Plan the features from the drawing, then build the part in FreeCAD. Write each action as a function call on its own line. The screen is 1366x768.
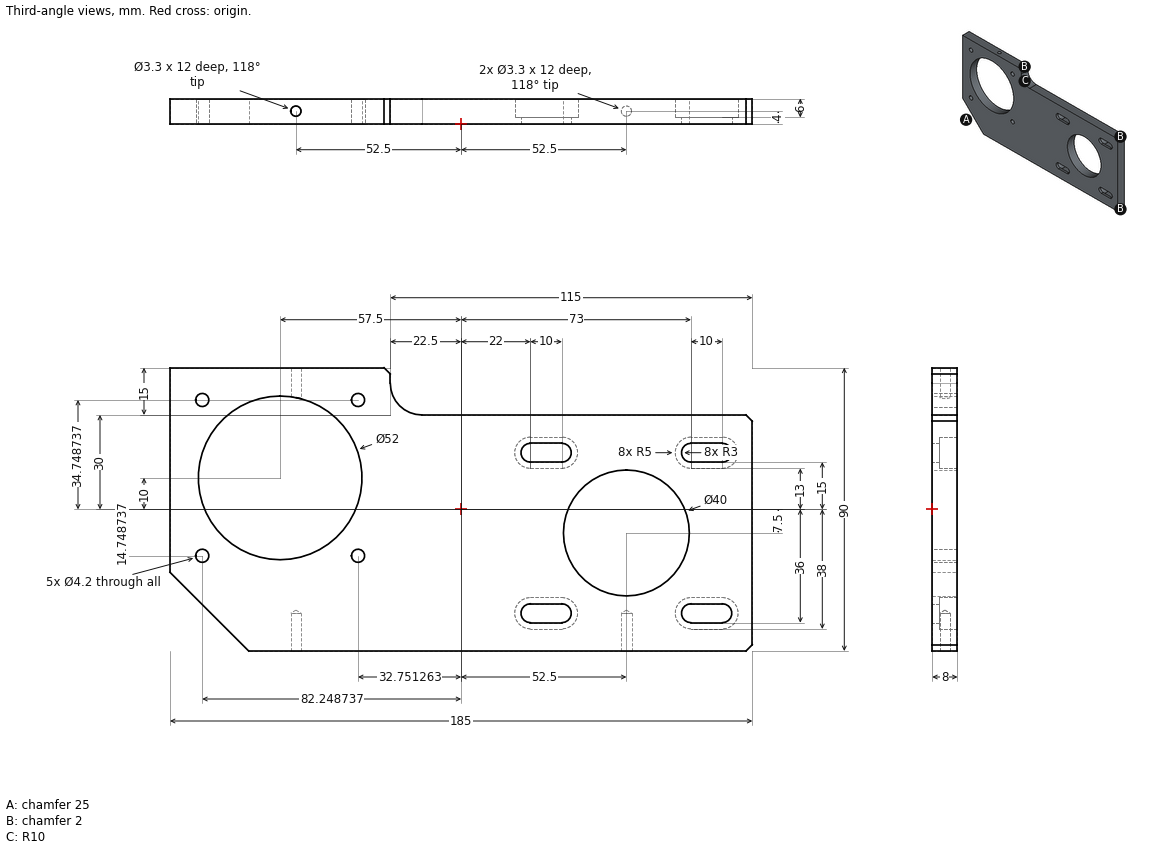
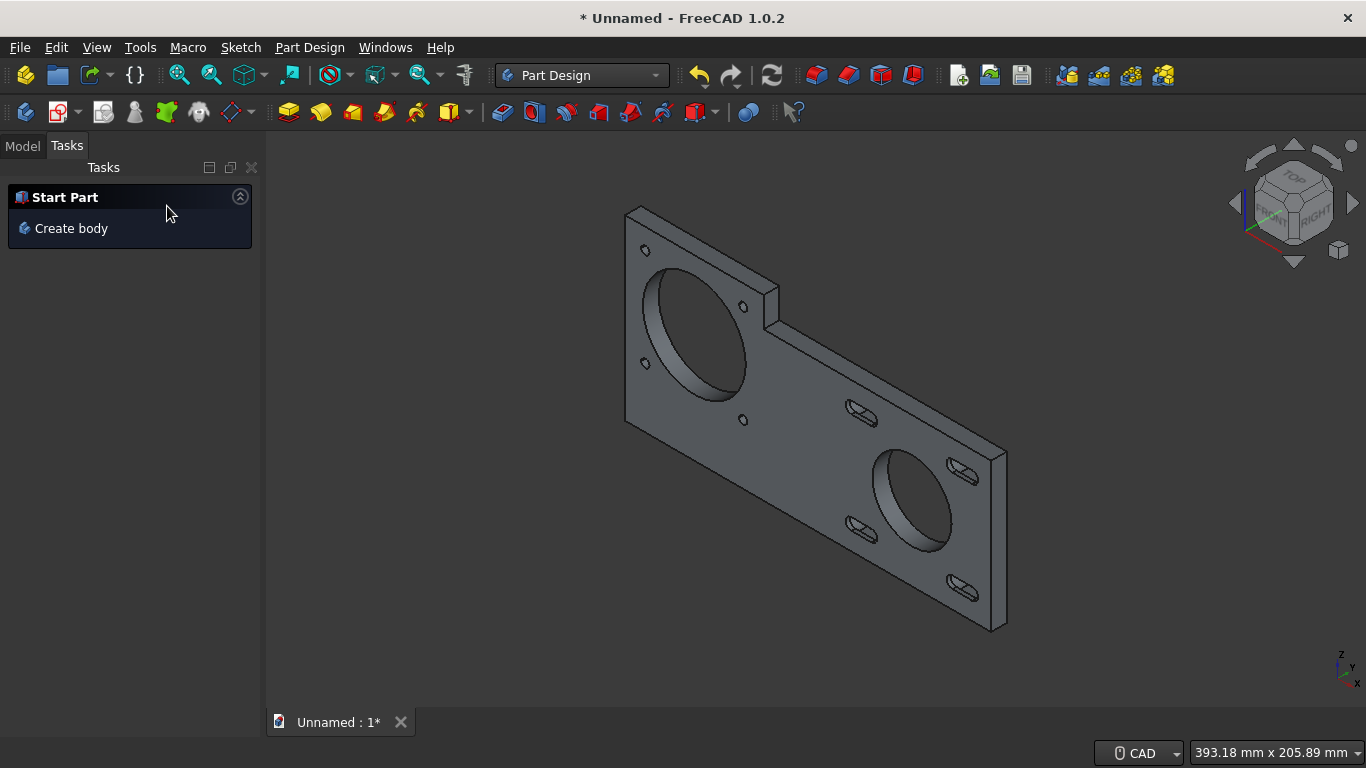
click(764, 282)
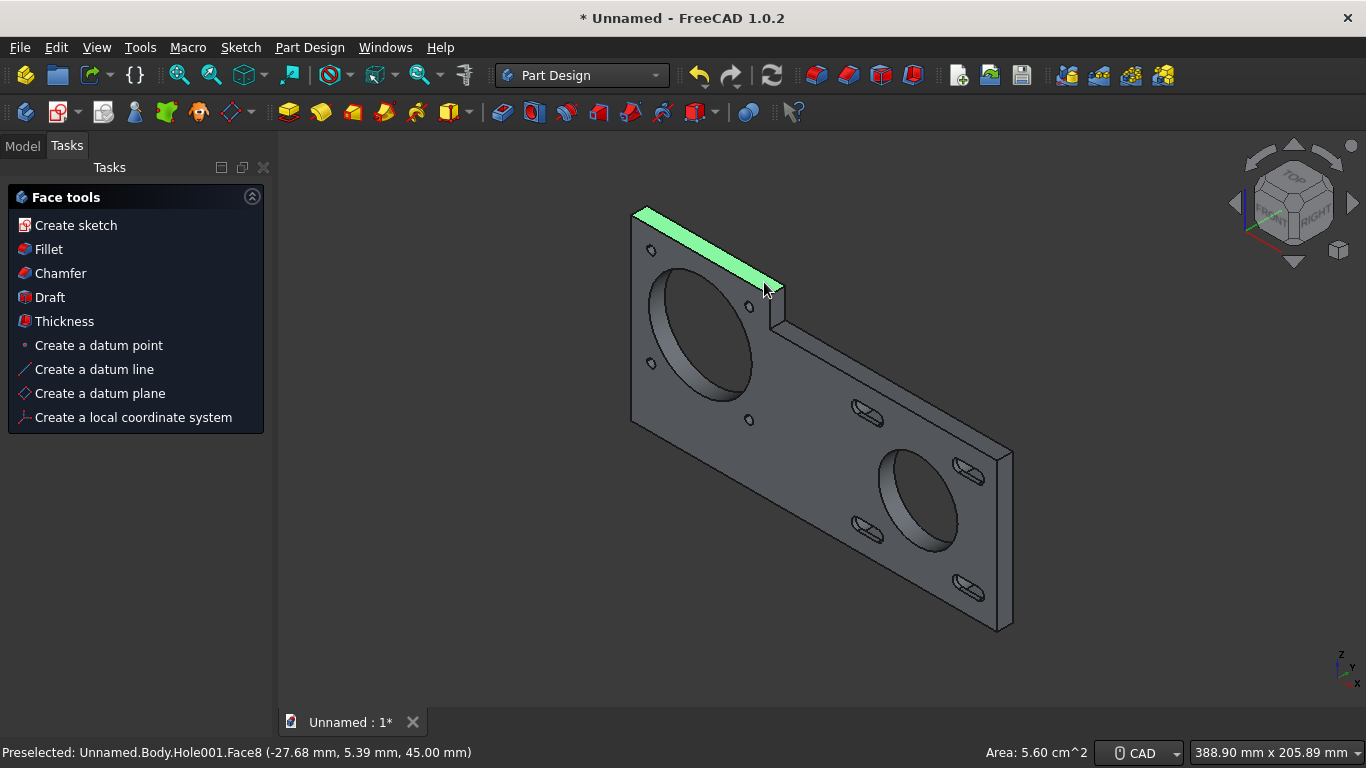
click(58, 112)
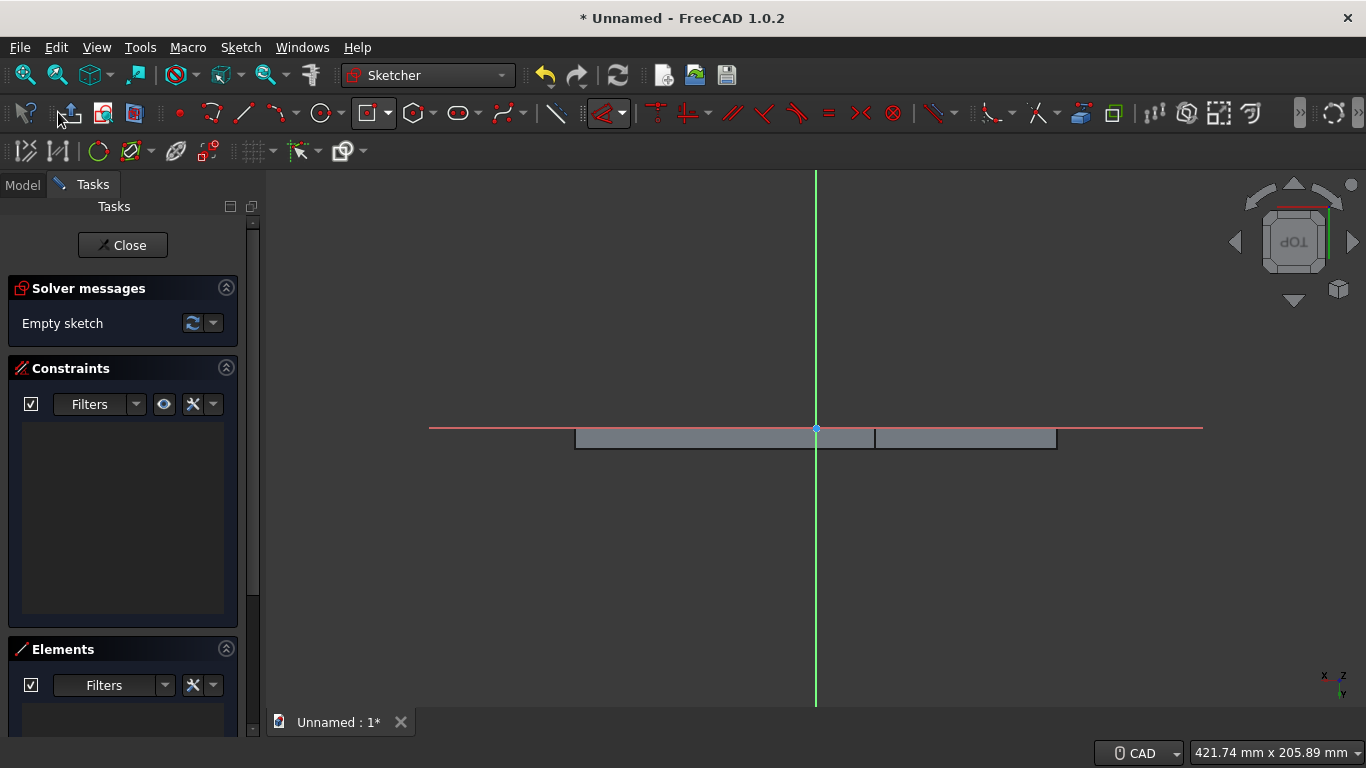
scroll(964, 439, up, 15)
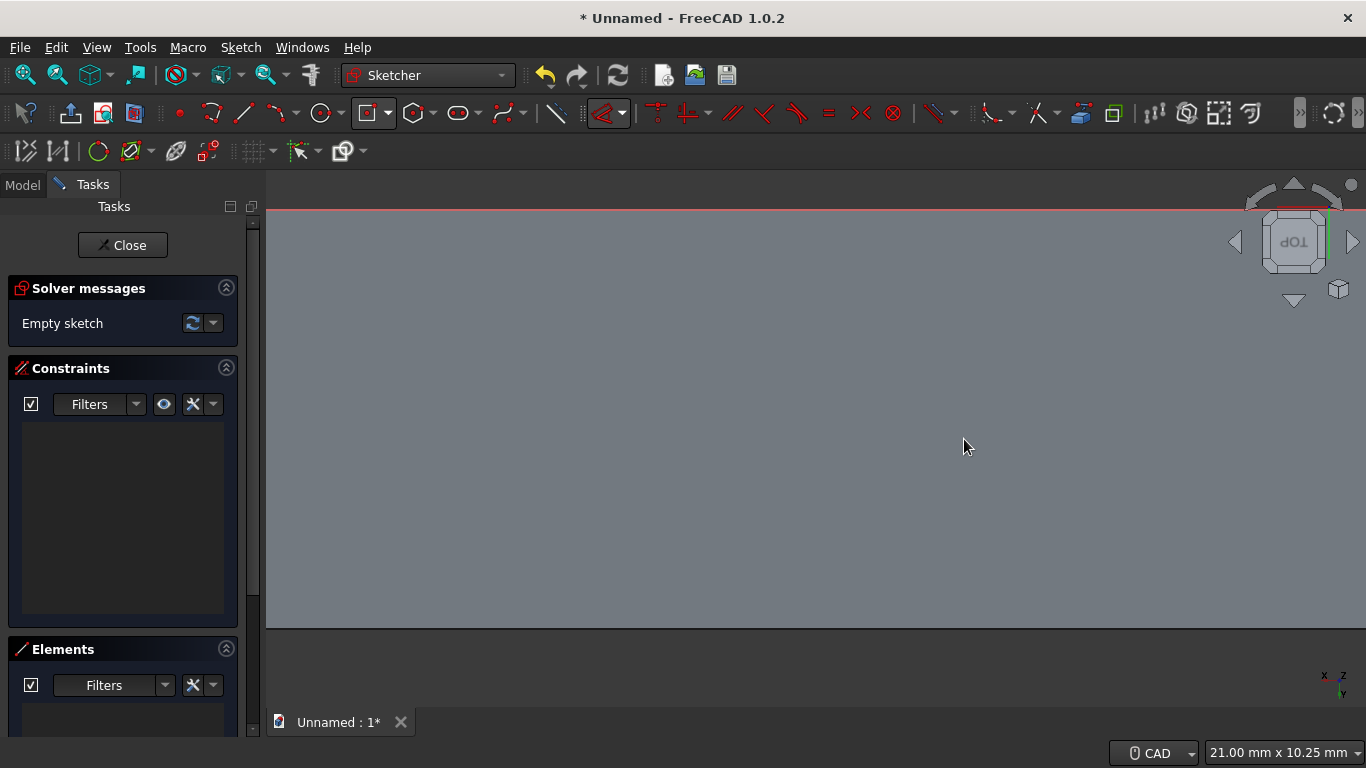
scroll(708, 396, up, 3)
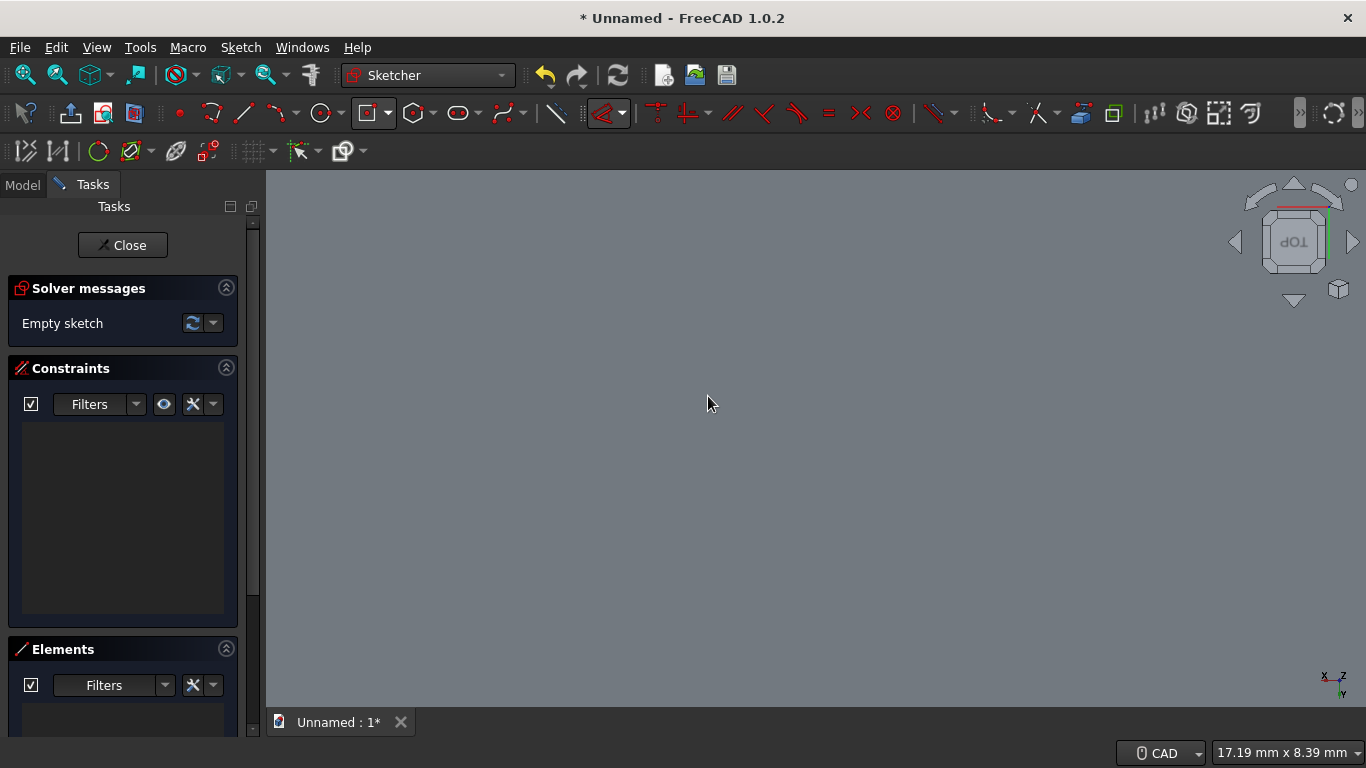
click(322, 114)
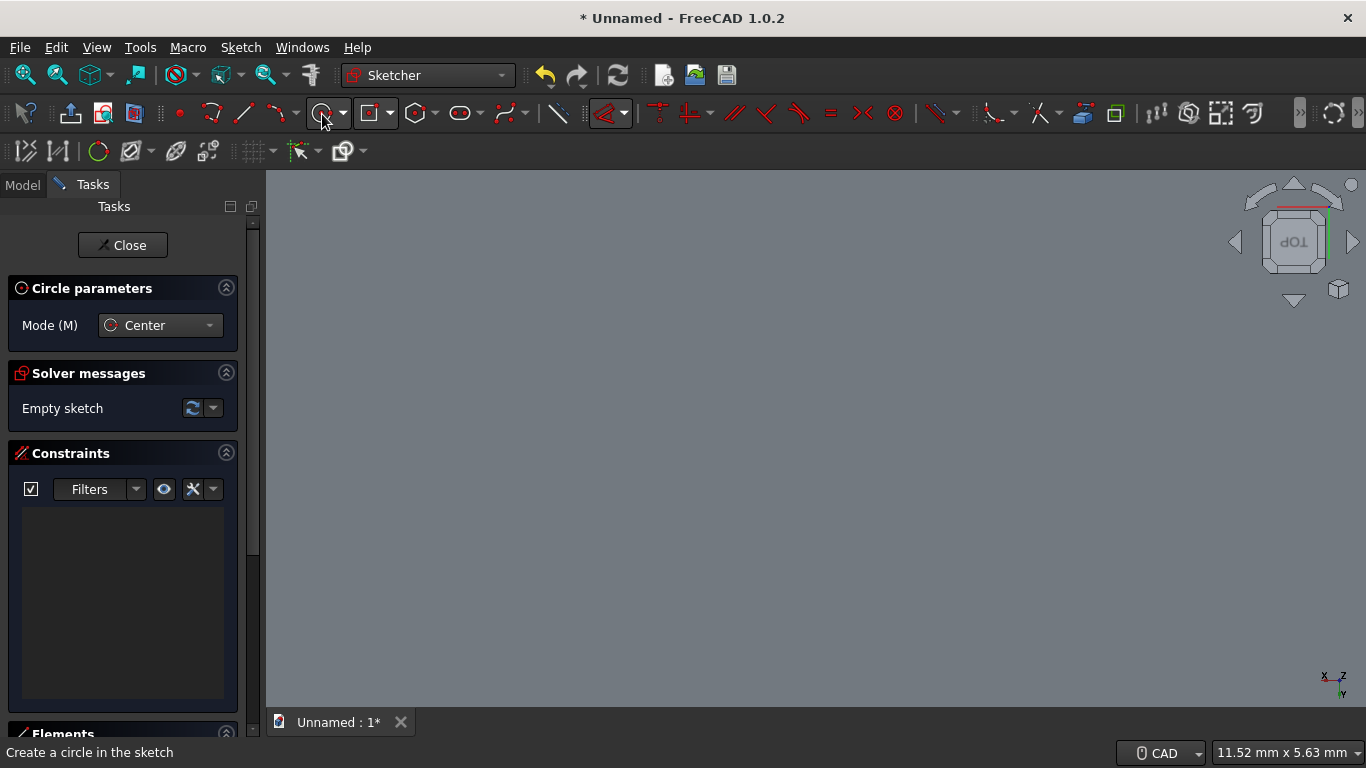
click(747, 438)
click(858, 327)
key(Escape)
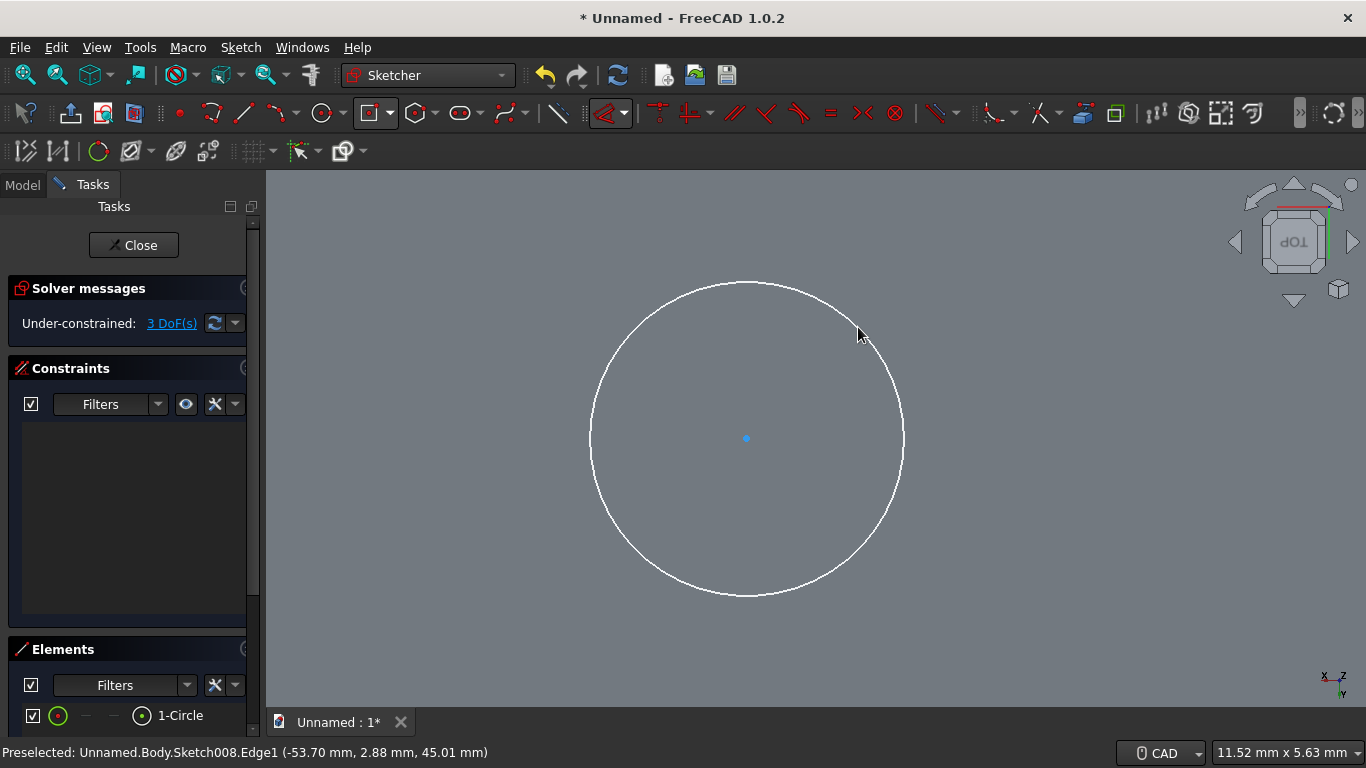
click(858, 328)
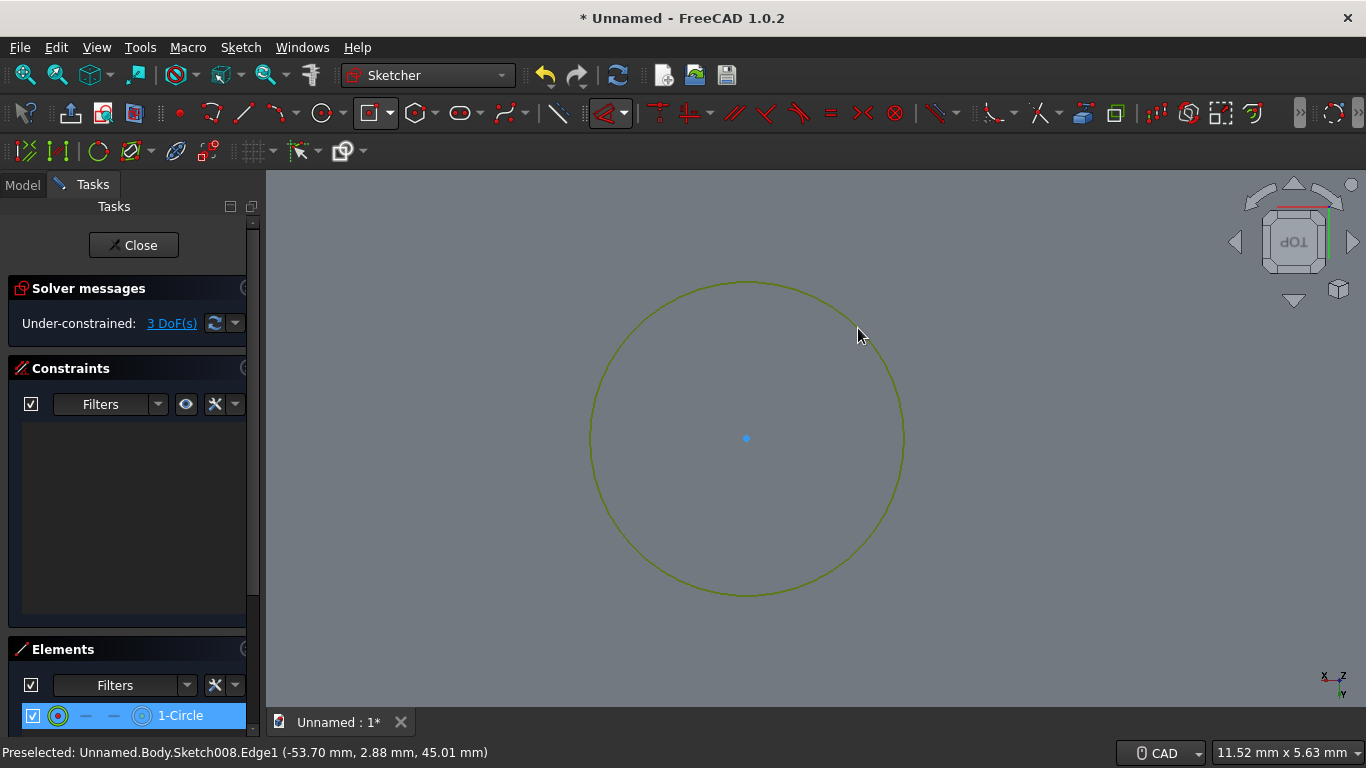
key(k)
key(o)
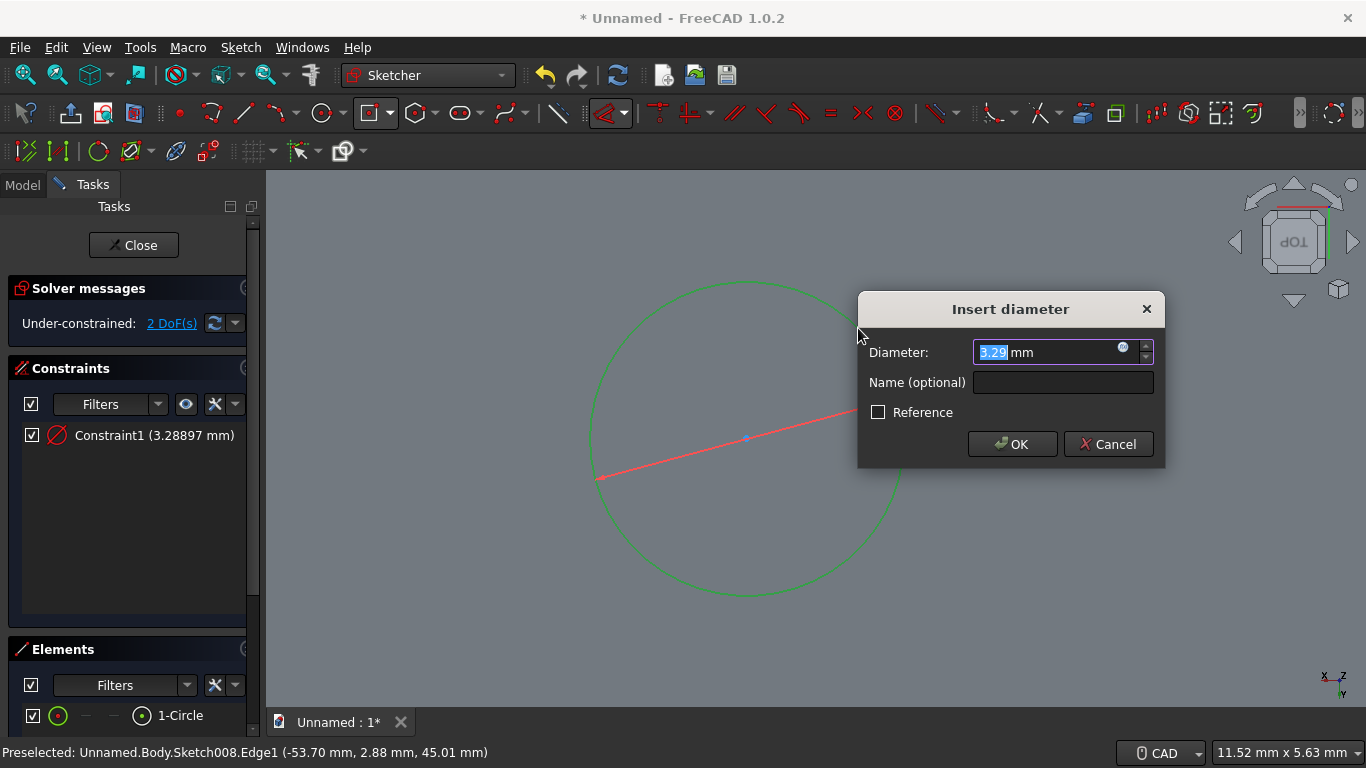
text(3.3)
key(Return)